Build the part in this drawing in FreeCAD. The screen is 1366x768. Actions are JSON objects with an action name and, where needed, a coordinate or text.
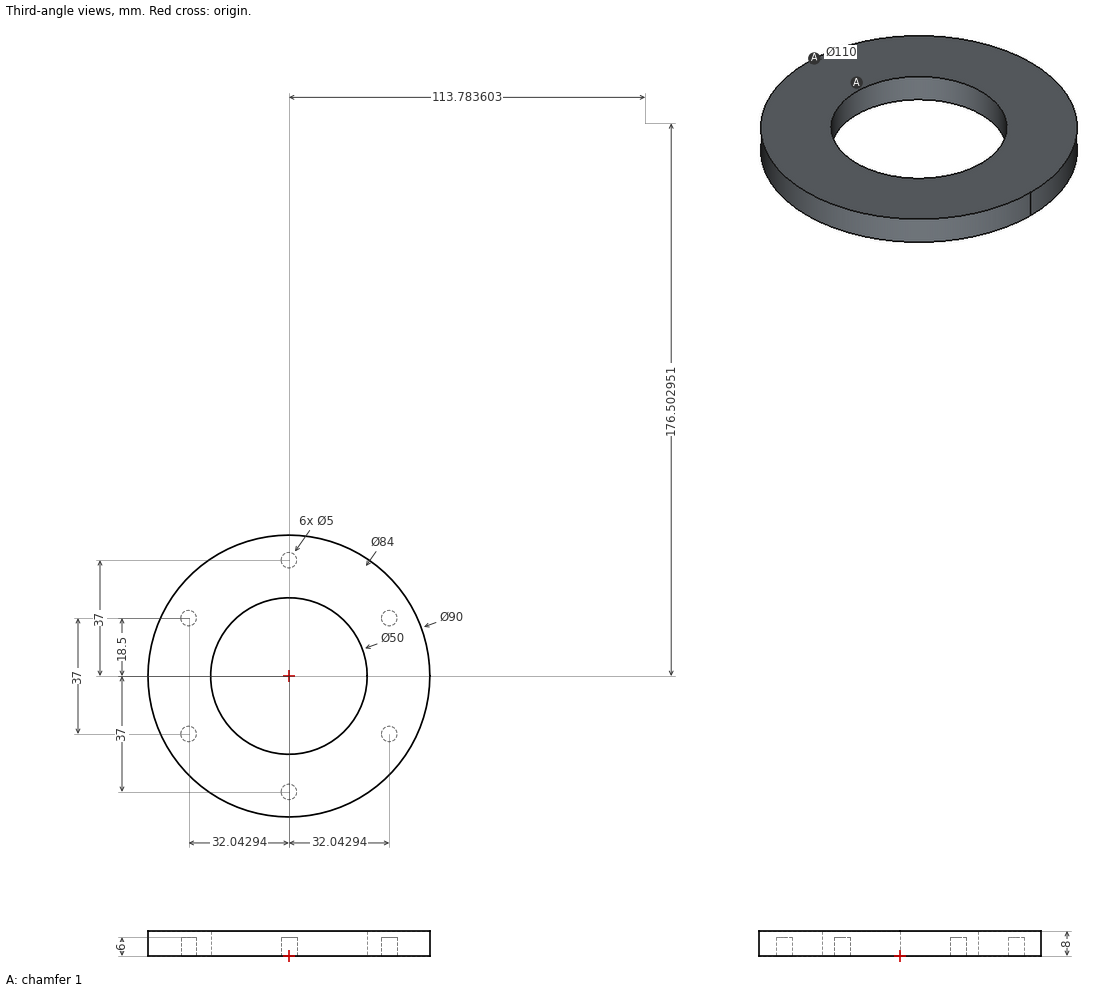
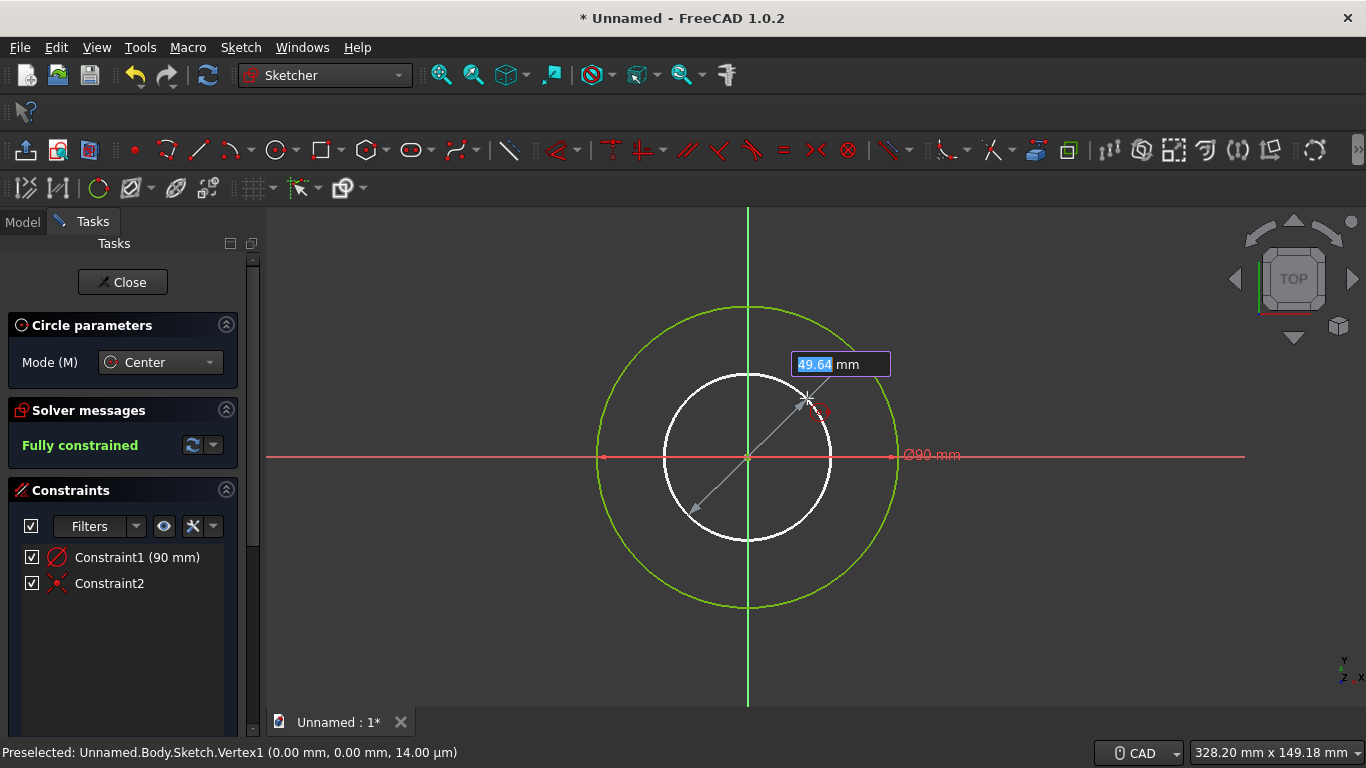
{"action": "type", "text": "50"}
{"action": "key", "text": "Return"}
{"action": "key", "text": "Escape"}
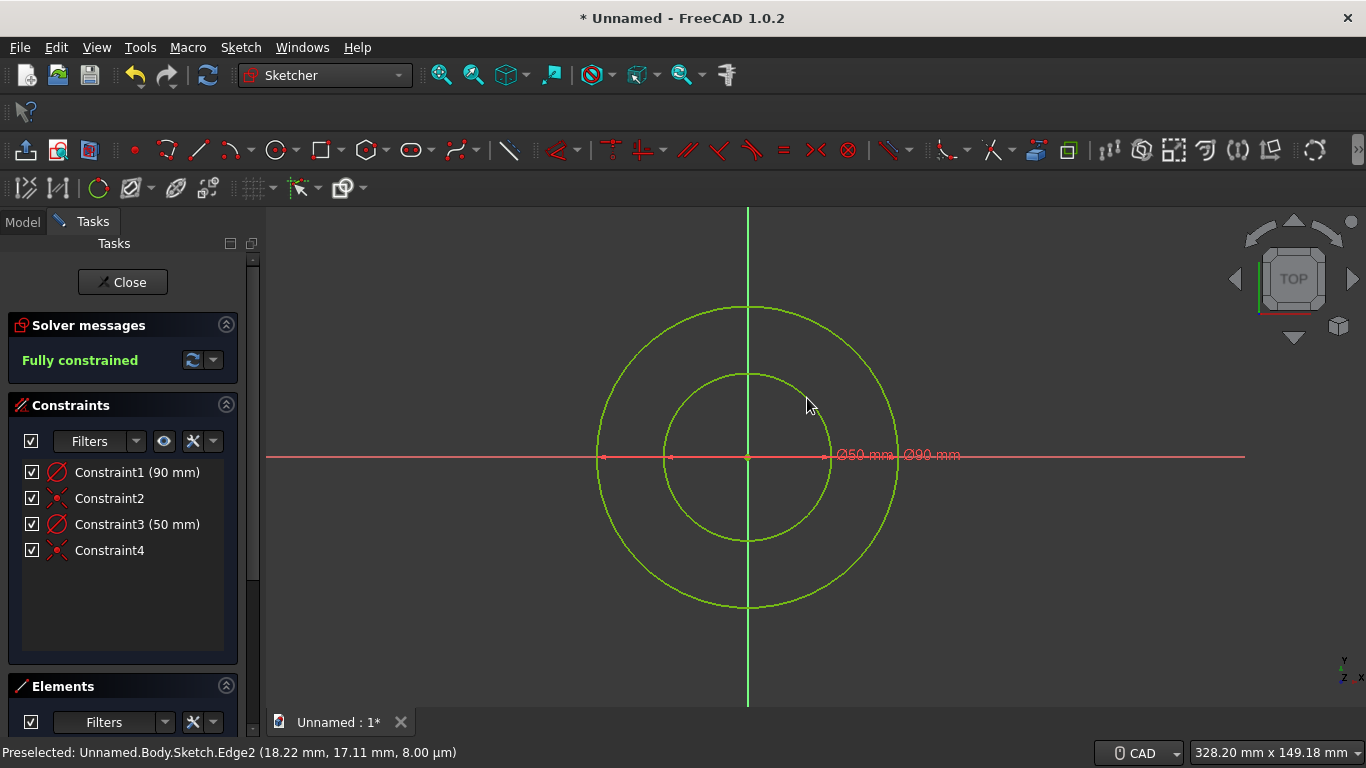
{"action": "left_click", "coordinate": [123, 282]}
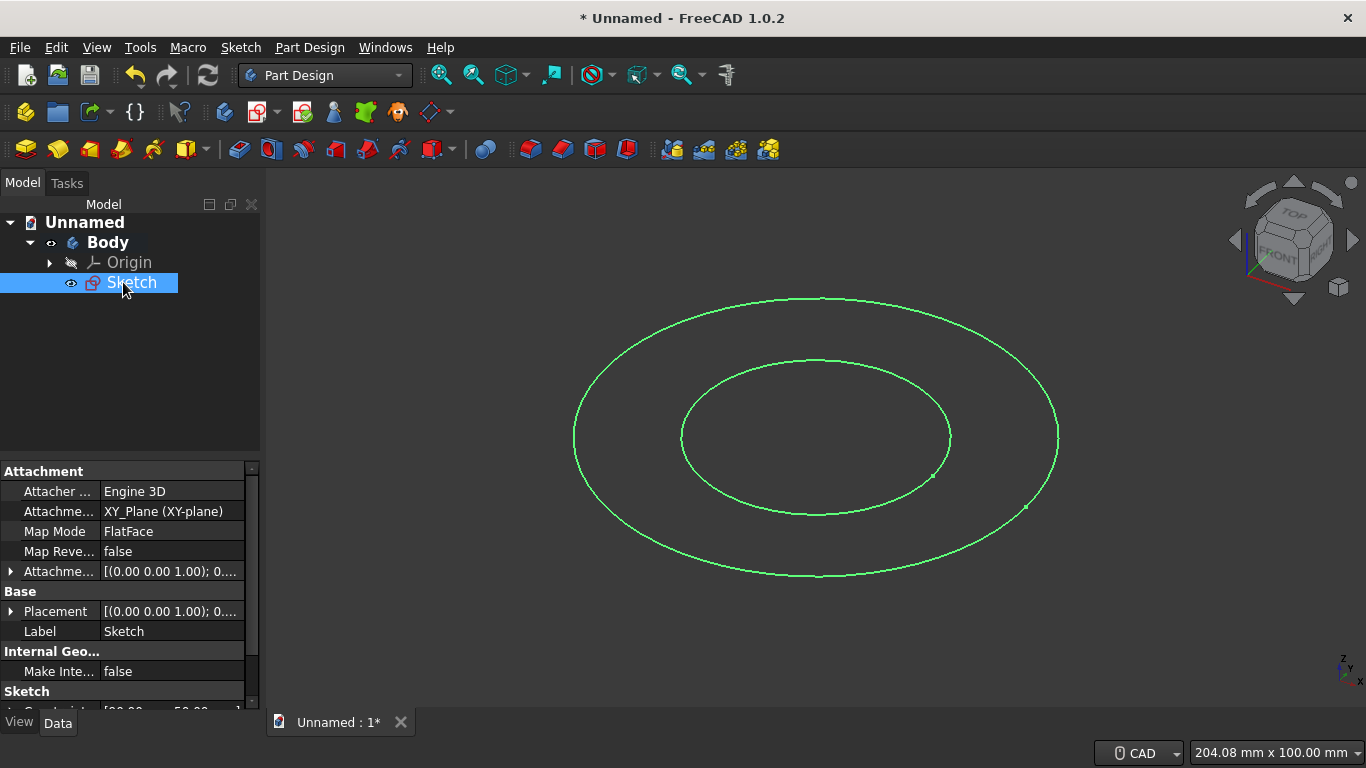
{"action": "left_click", "coordinate": [26, 150]}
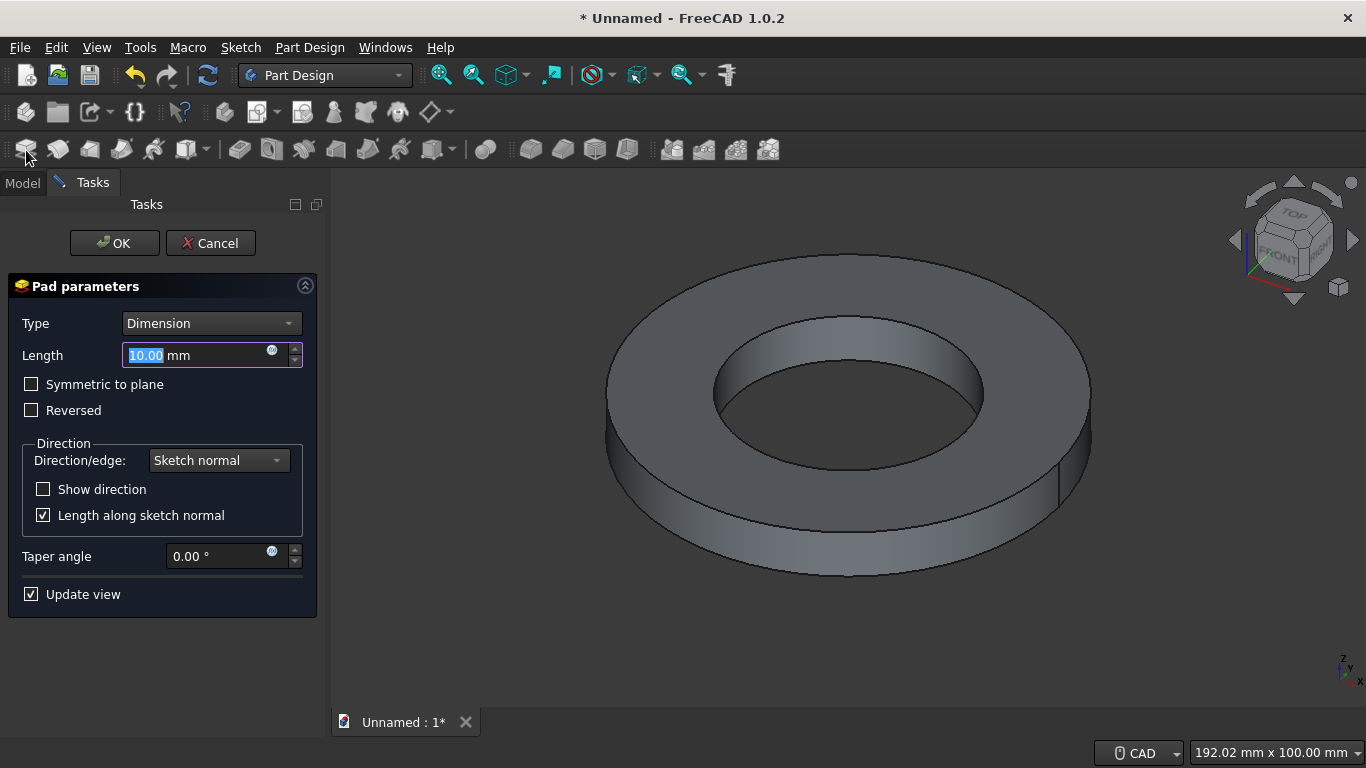
{"action": "type", "text": "8"}
{"action": "key", "text": "Tab"}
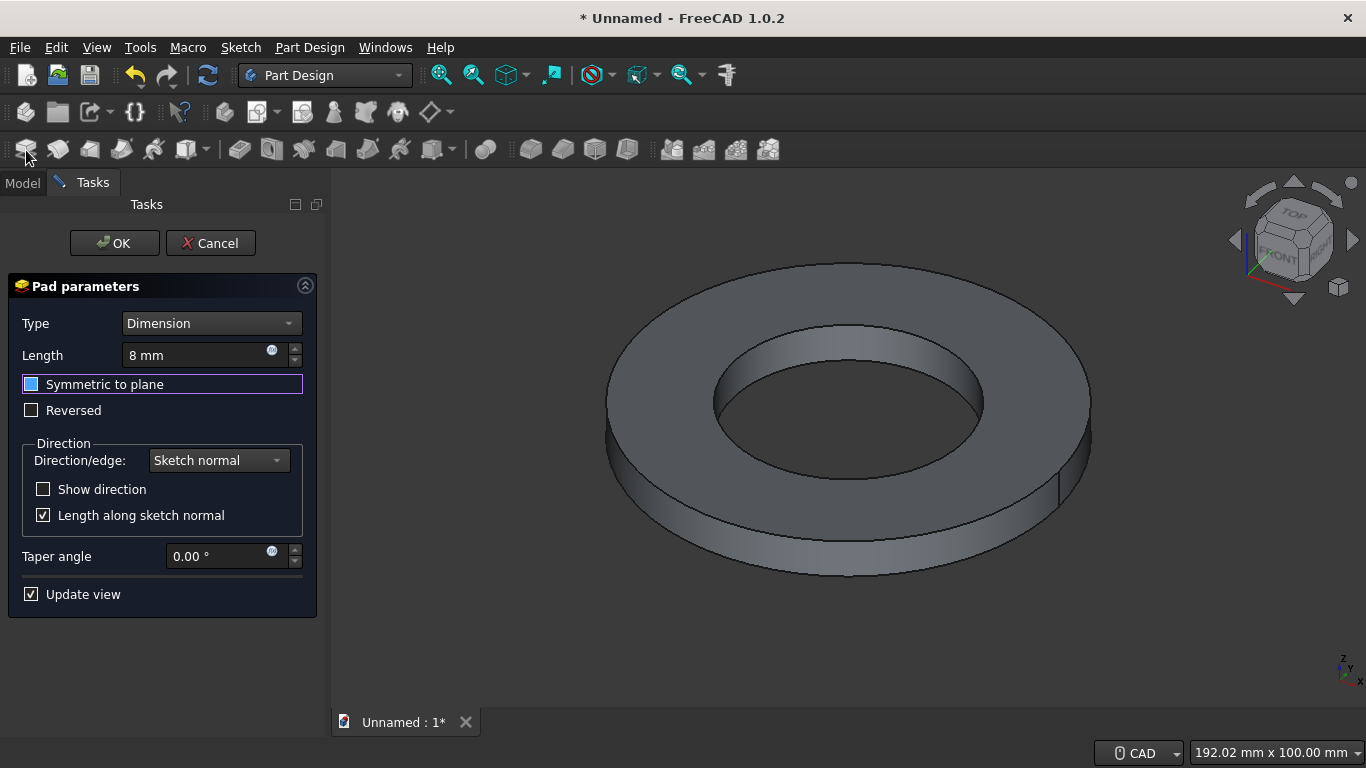
{"action": "left_click", "coordinate": [115, 243]}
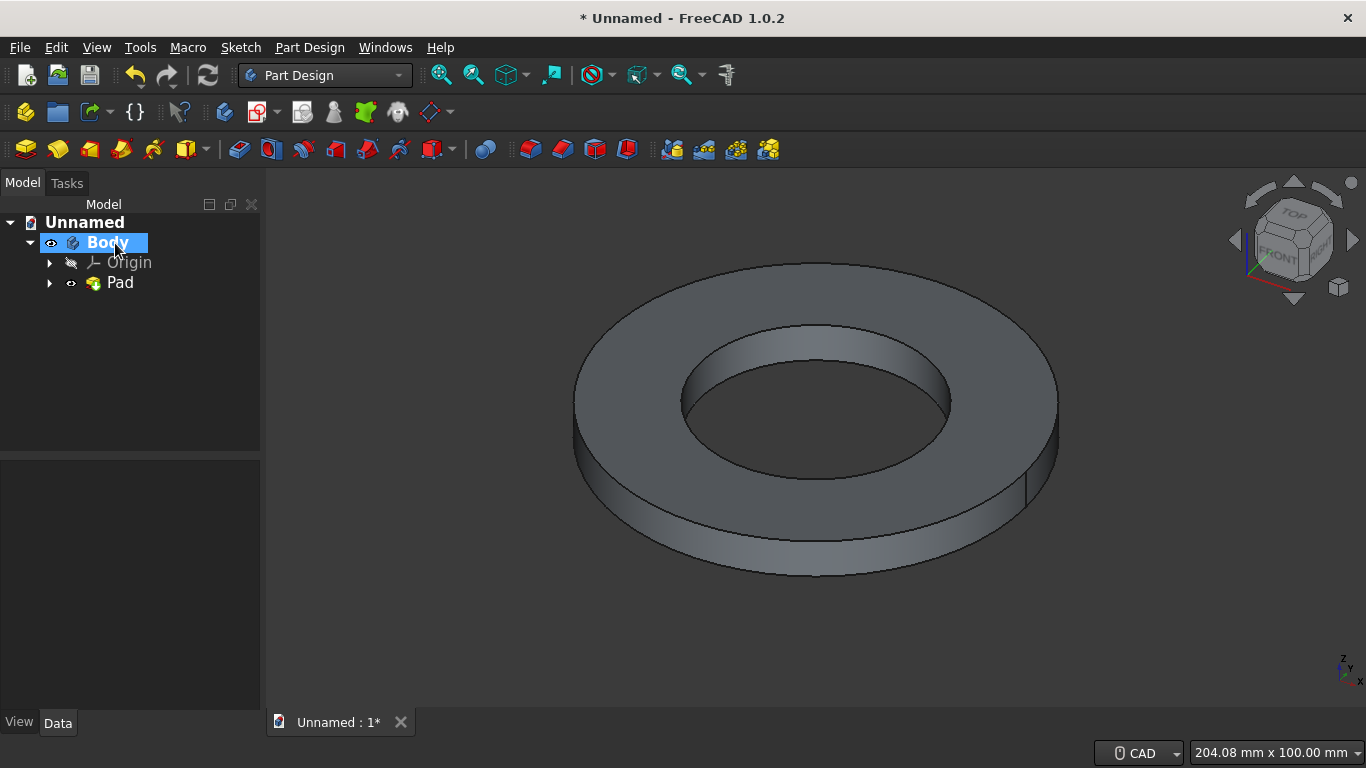
{"action": "left_click", "coordinate": [1005, 372]}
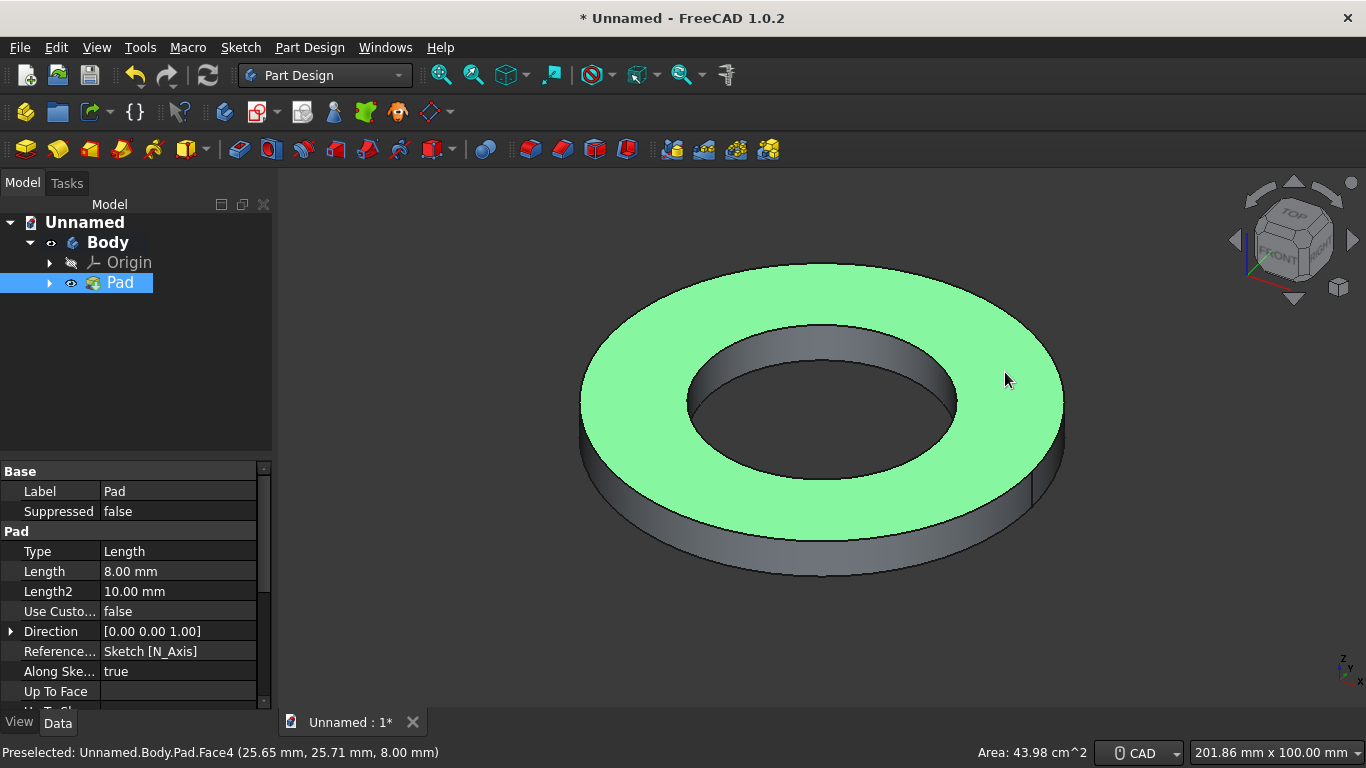
{"action": "left_click", "coordinate": [258, 112]}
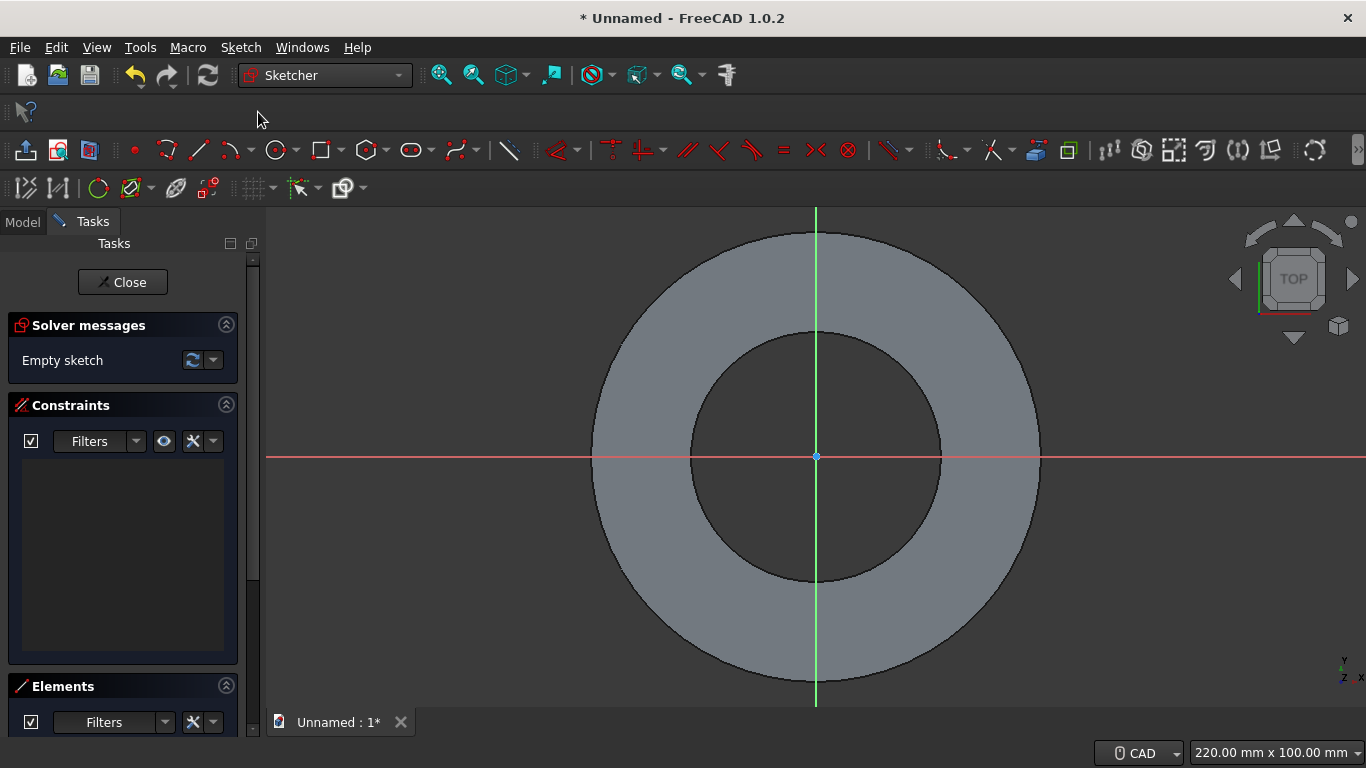
{"action": "scroll", "coordinate": [438, 457], "scroll_direction": "down", "scroll_amount": 1}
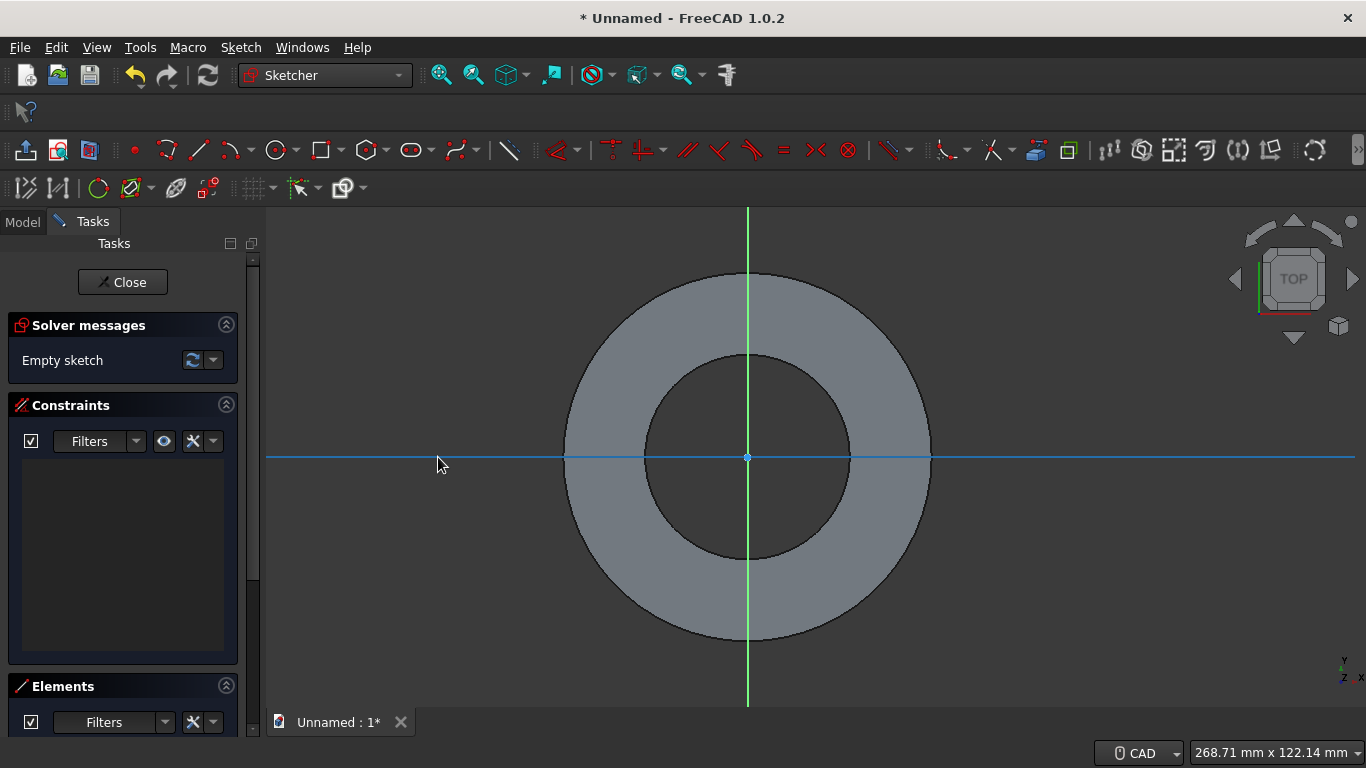
{"action": "key", "text": "g c"}